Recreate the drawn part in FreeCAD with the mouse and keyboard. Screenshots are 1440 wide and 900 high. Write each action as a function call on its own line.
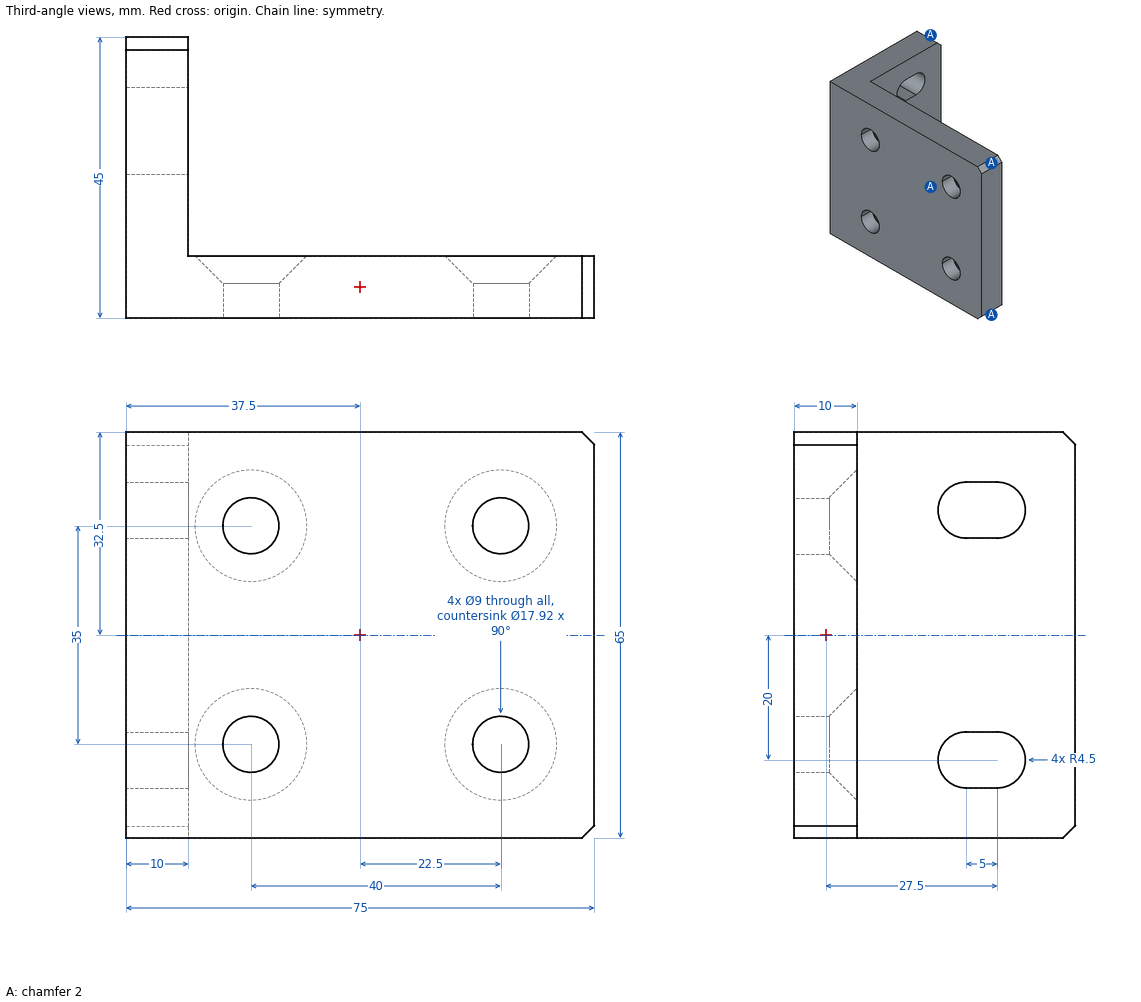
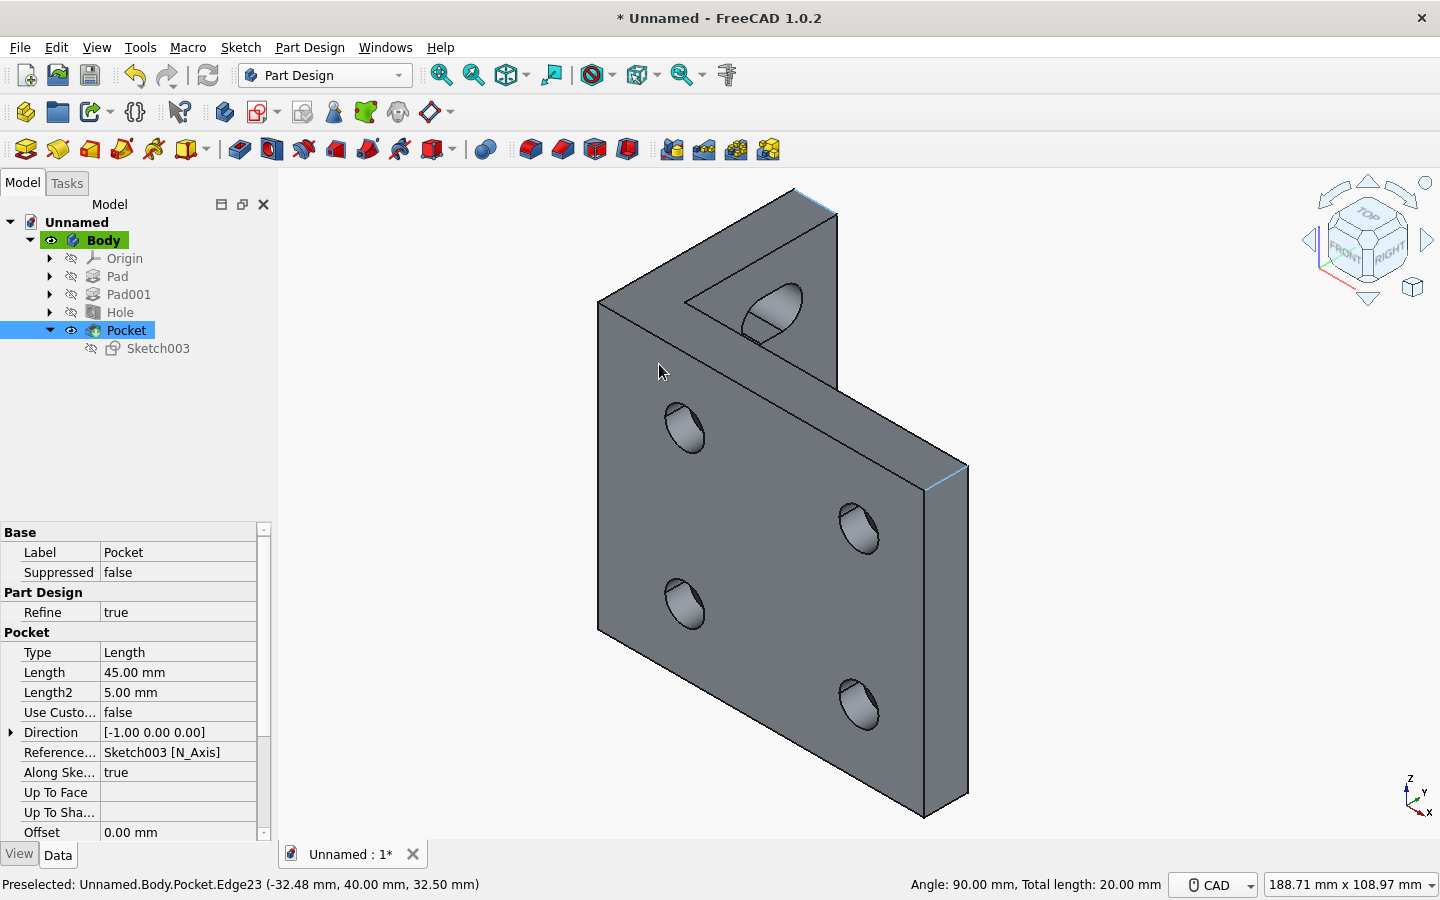
key(1)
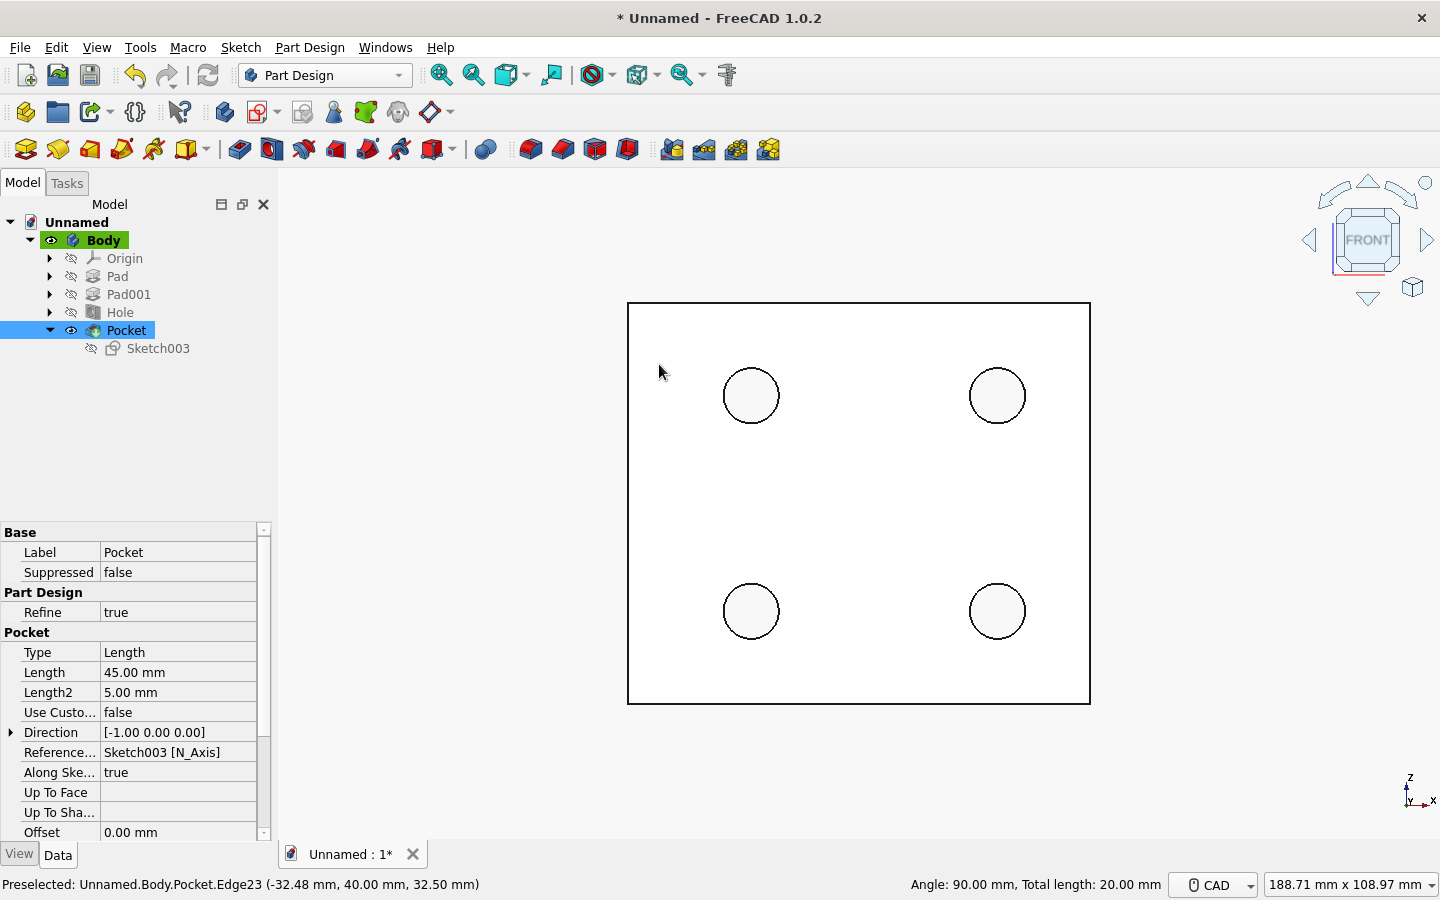
key(3)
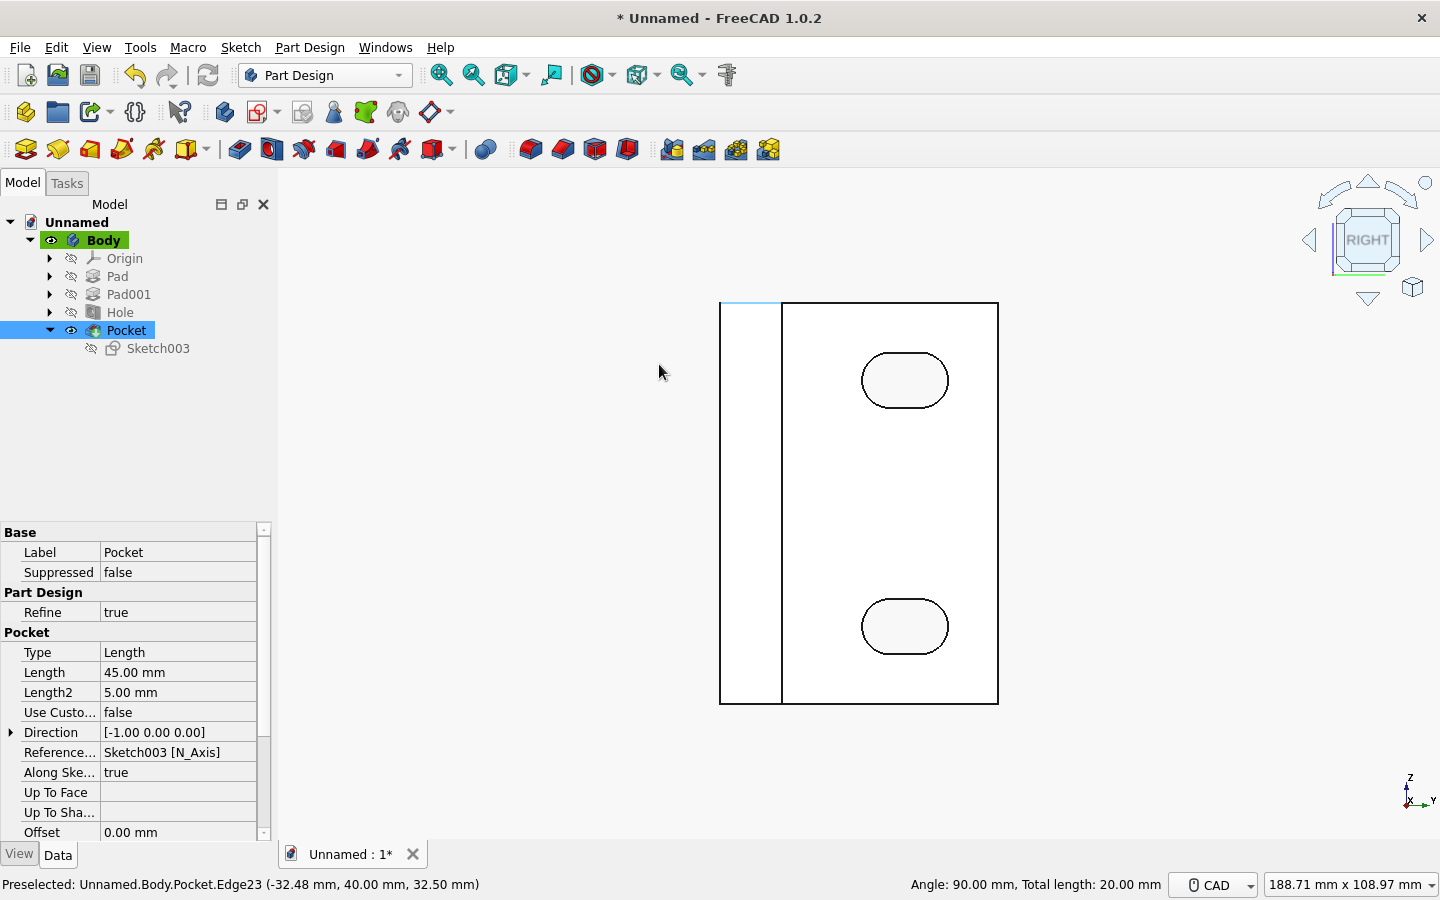
click(751, 703, ctrl)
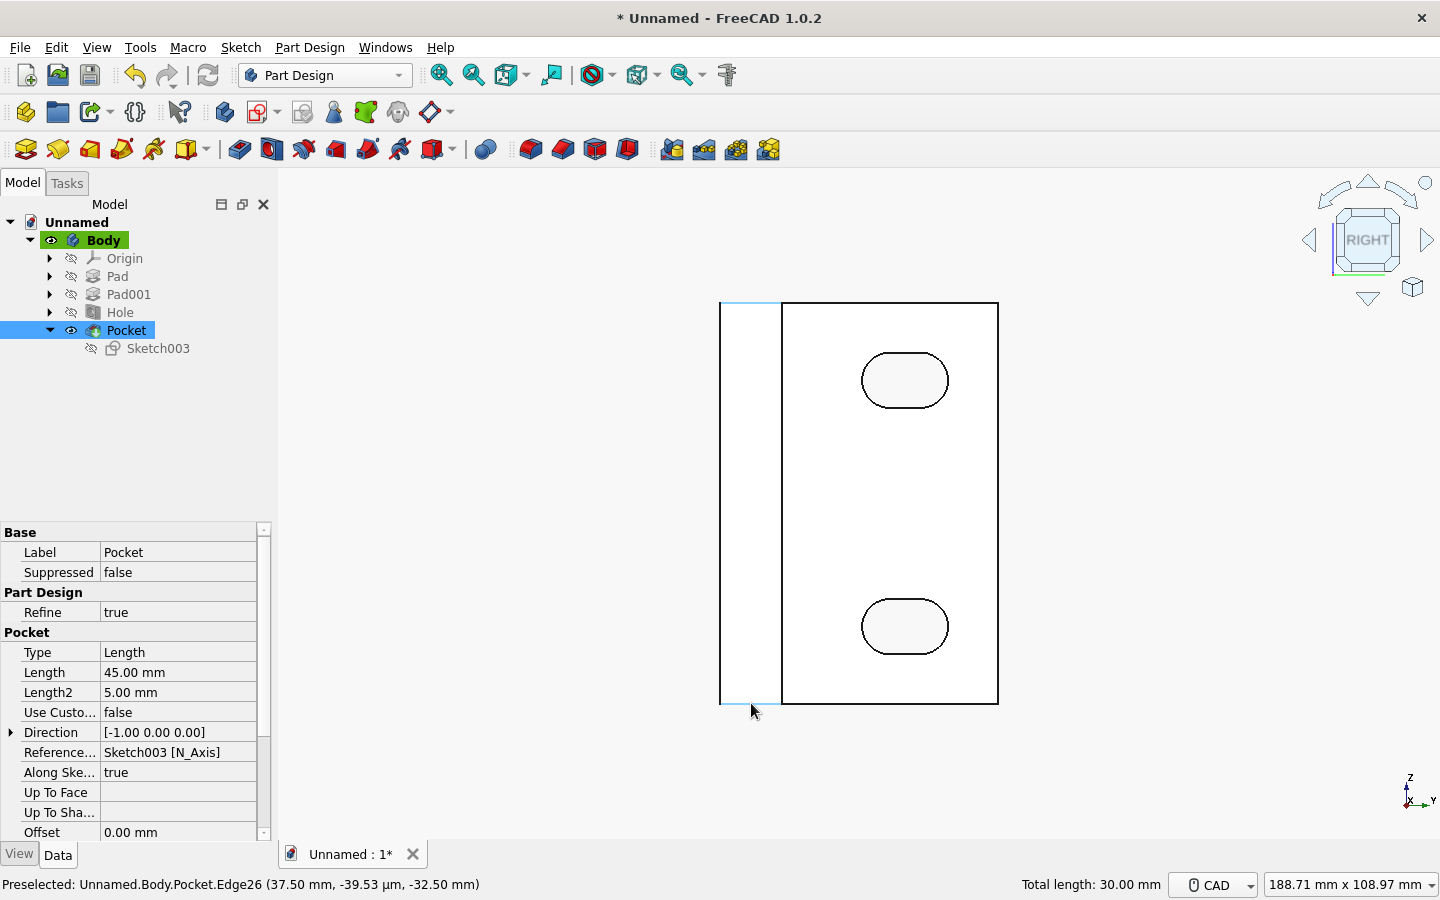
key(5)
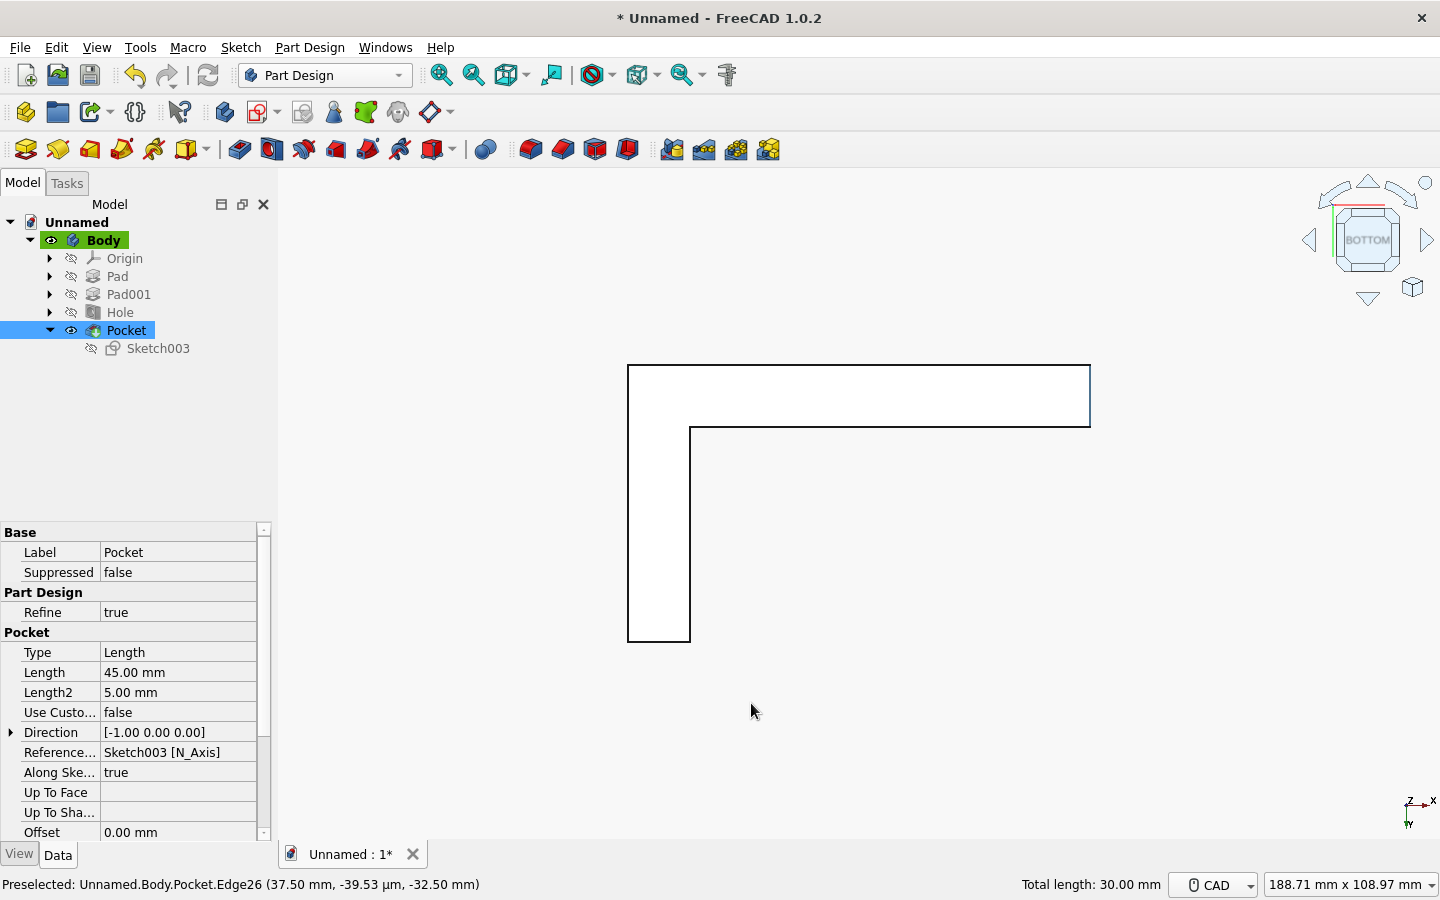
key(v)
key(f)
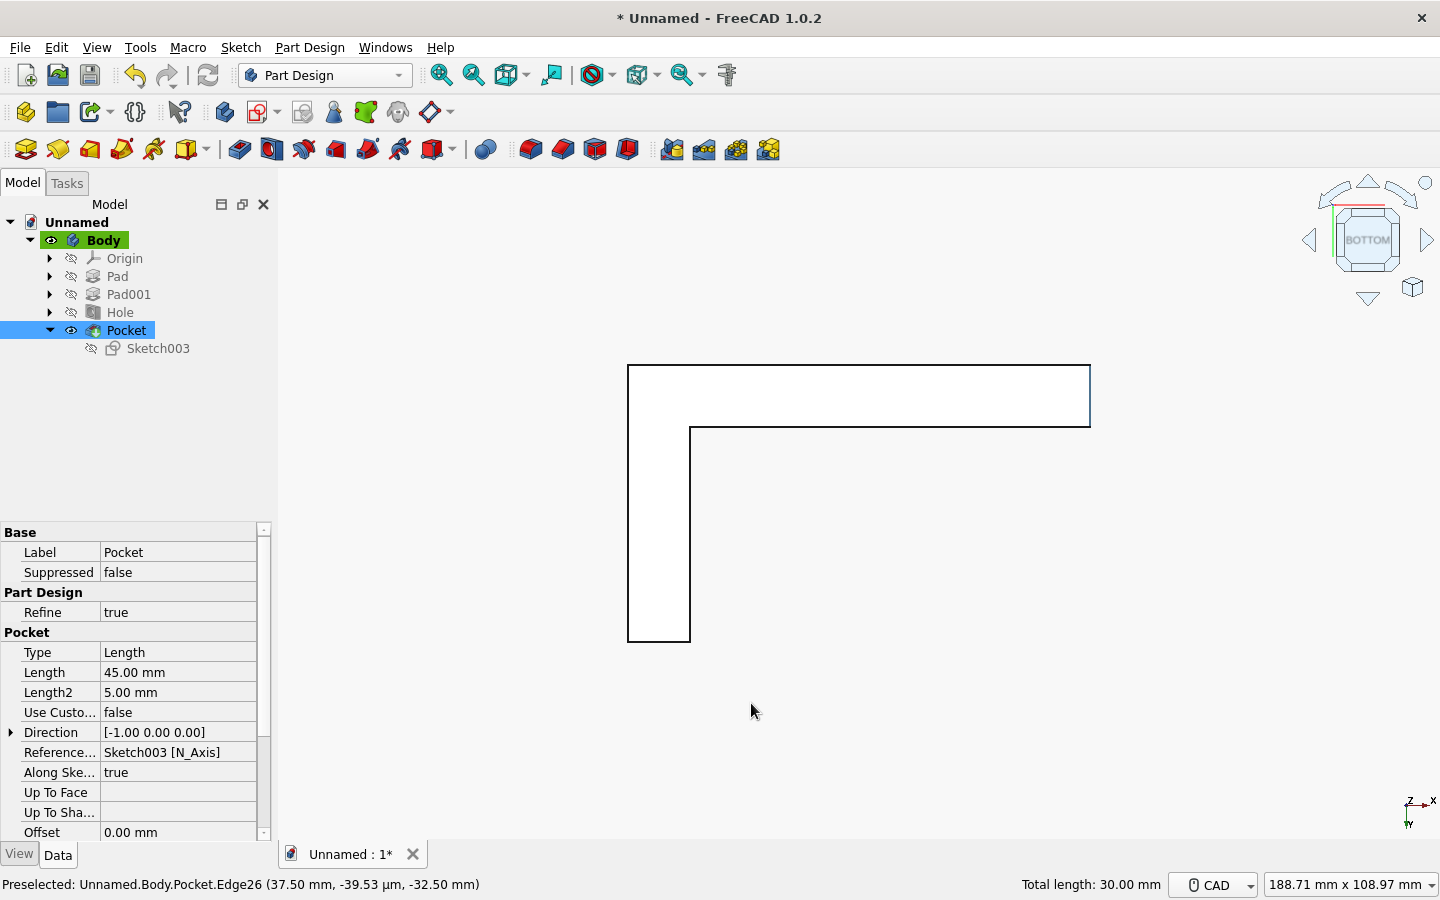
key(4)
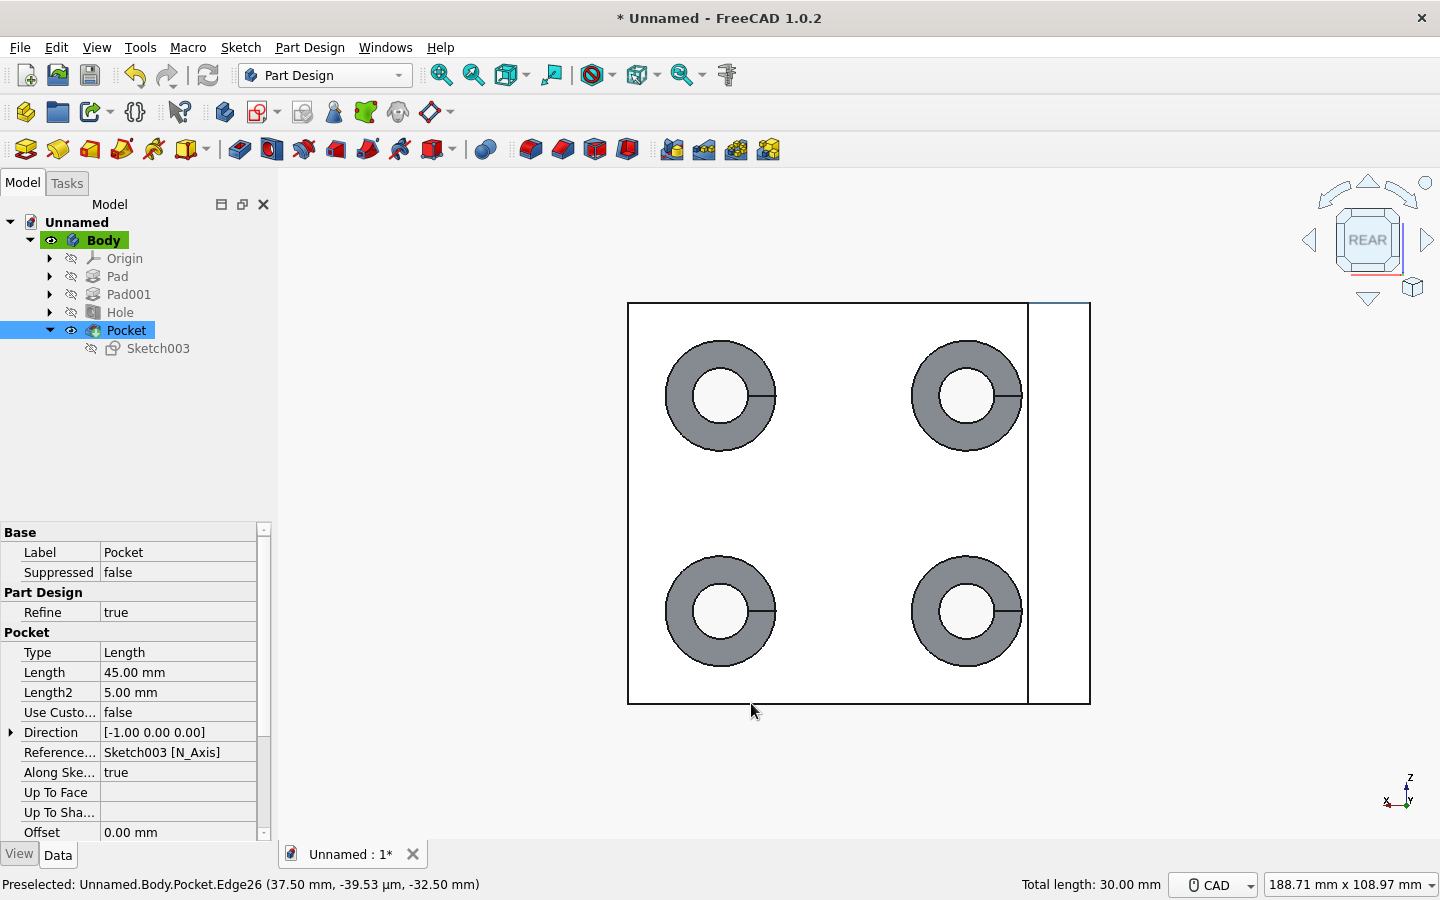
click(1059, 703, ctrl)